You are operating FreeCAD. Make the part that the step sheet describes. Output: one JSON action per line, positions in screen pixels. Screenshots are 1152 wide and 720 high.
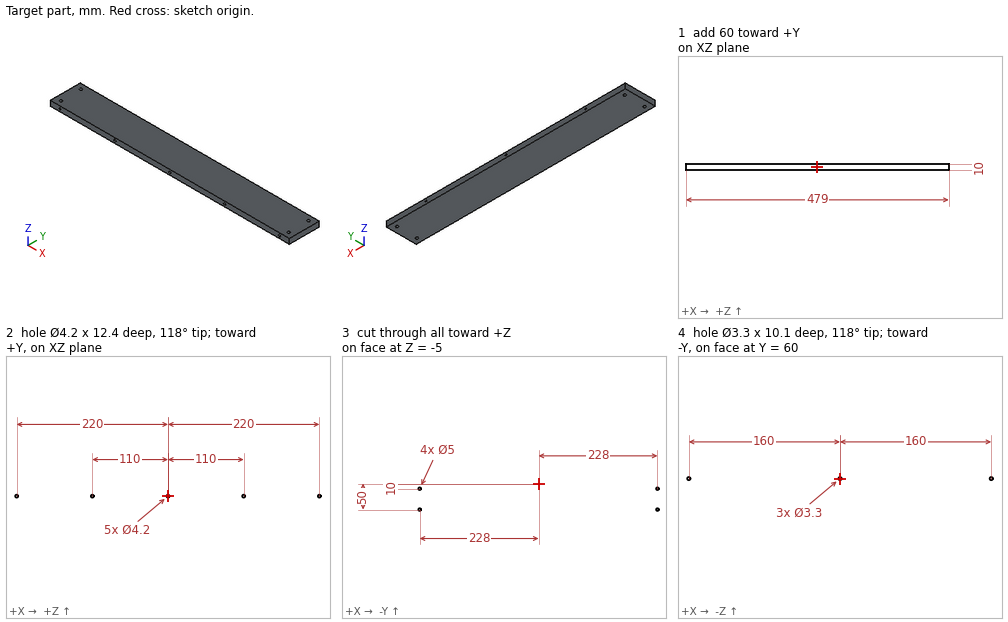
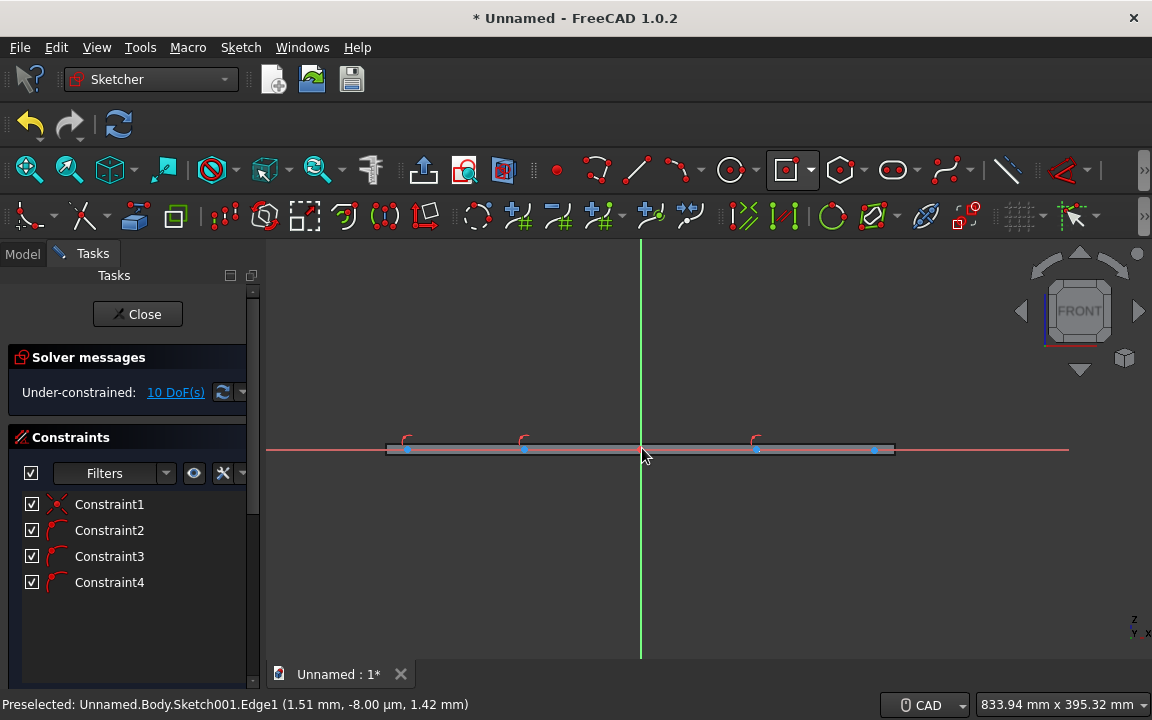
{"action": "scroll", "coordinate": [759, 448], "scroll_direction": "up", "scroll_amount": 11}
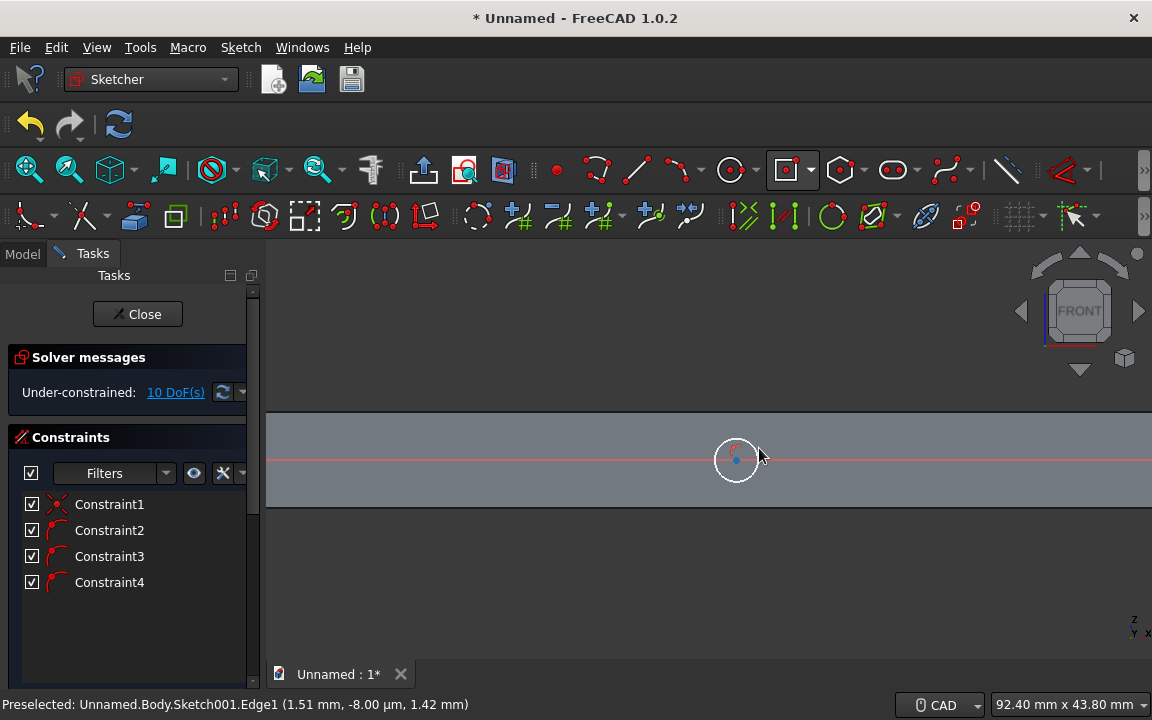
{"action": "left_click", "coordinate": [752, 445]}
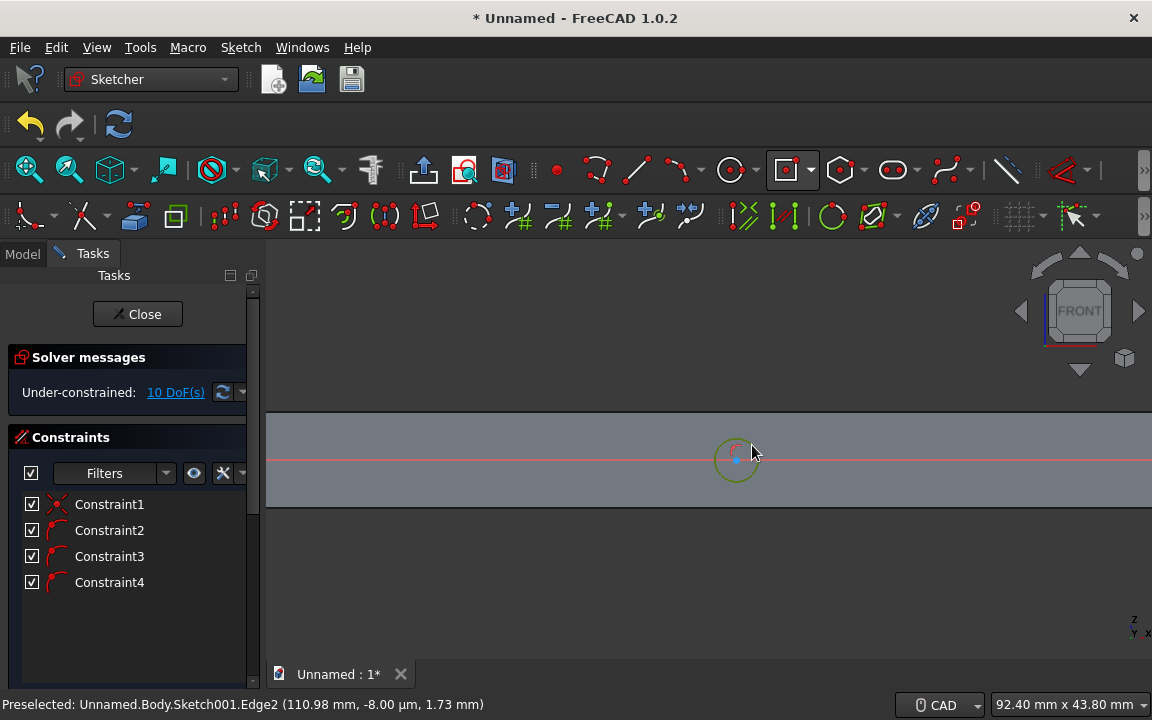
{"action": "scroll", "coordinate": [759, 448], "scroll_direction": "down", "scroll_amount": 11}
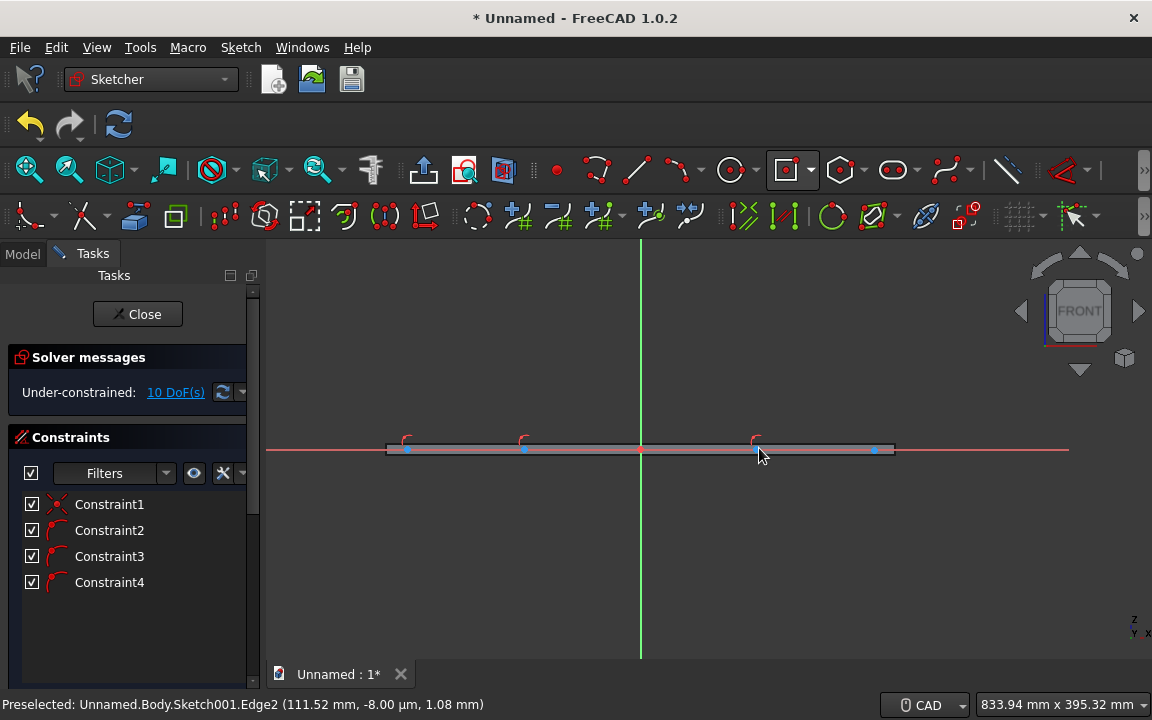
{"action": "scroll", "coordinate": [875, 450], "scroll_direction": "up", "scroll_amount": 13}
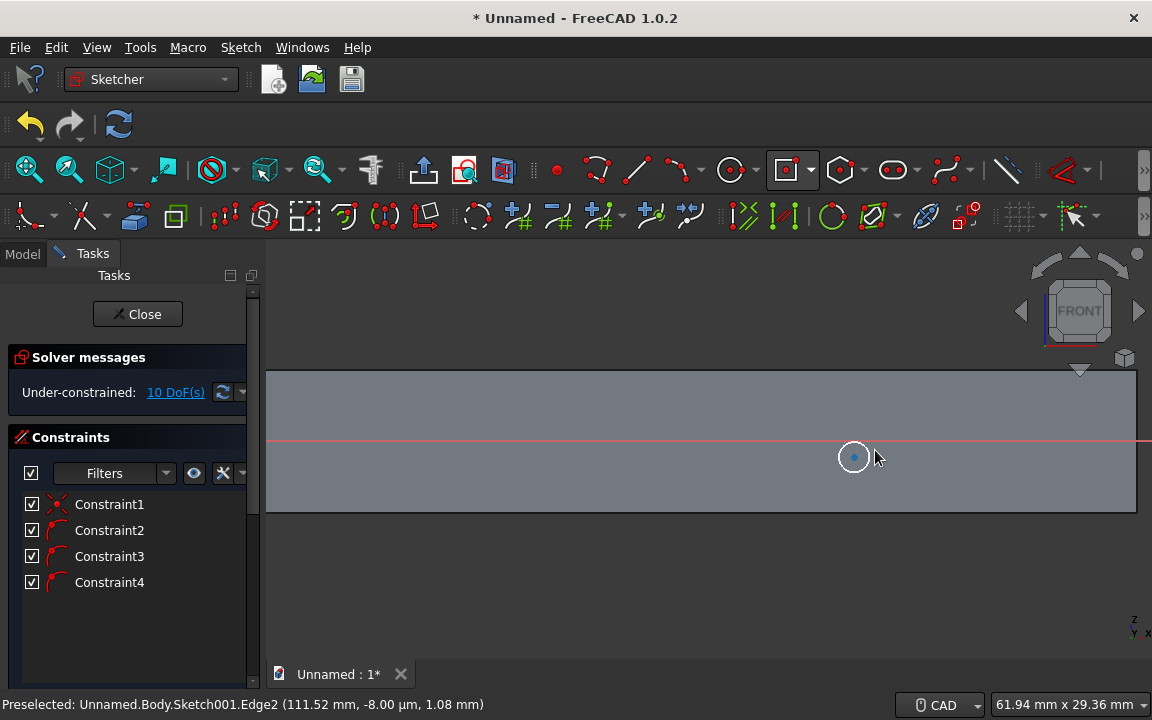
{"action": "left_click", "coordinate": [865, 446]}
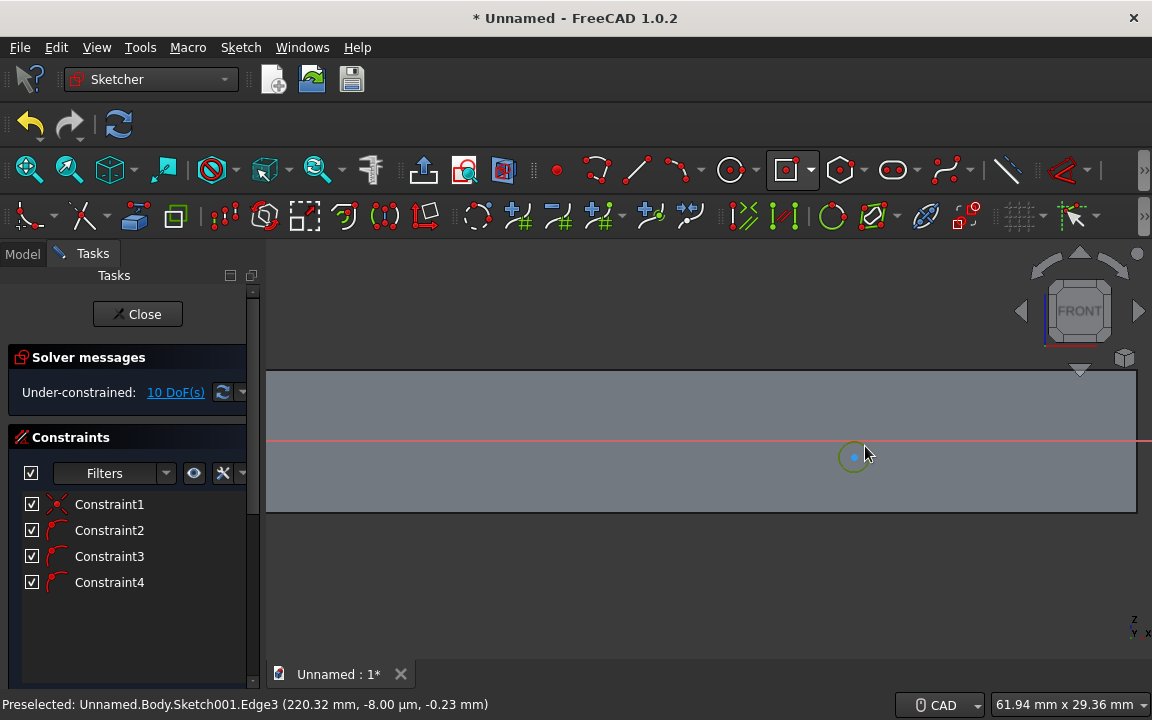
{"action": "scroll", "coordinate": [876, 450], "scroll_direction": "down", "scroll_amount": 13}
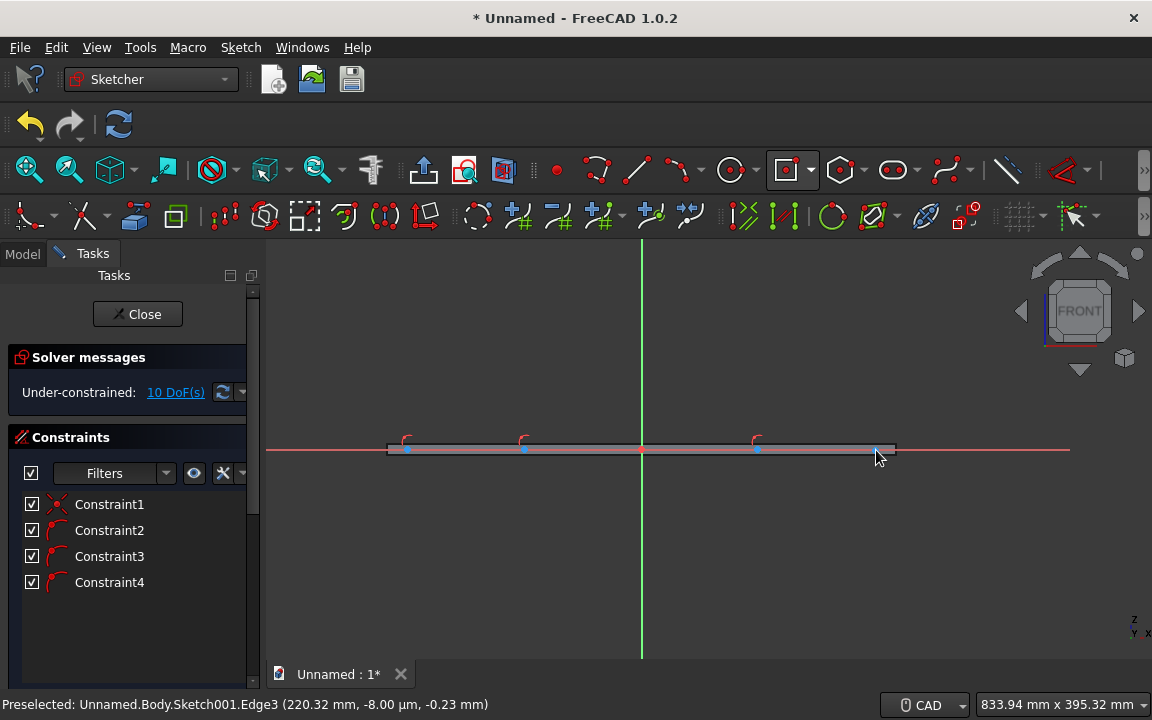
{"action": "scroll", "coordinate": [409, 448], "scroll_direction": "up", "scroll_amount": 12}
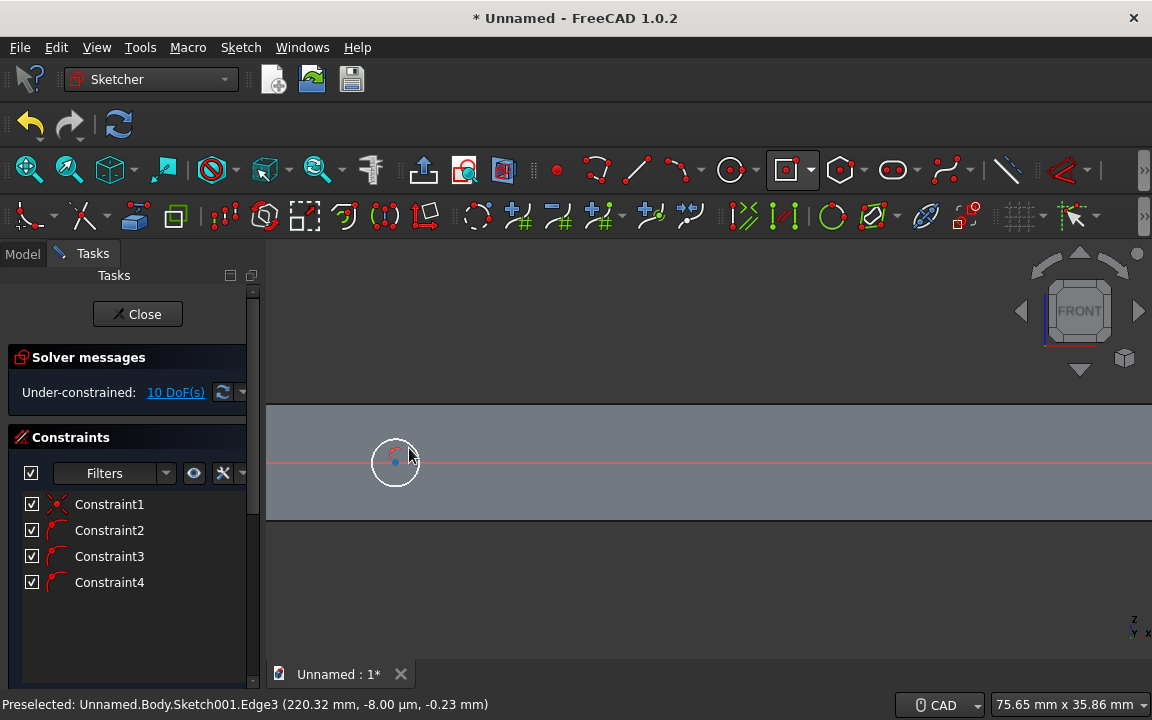
{"action": "left_click", "coordinate": [412, 446]}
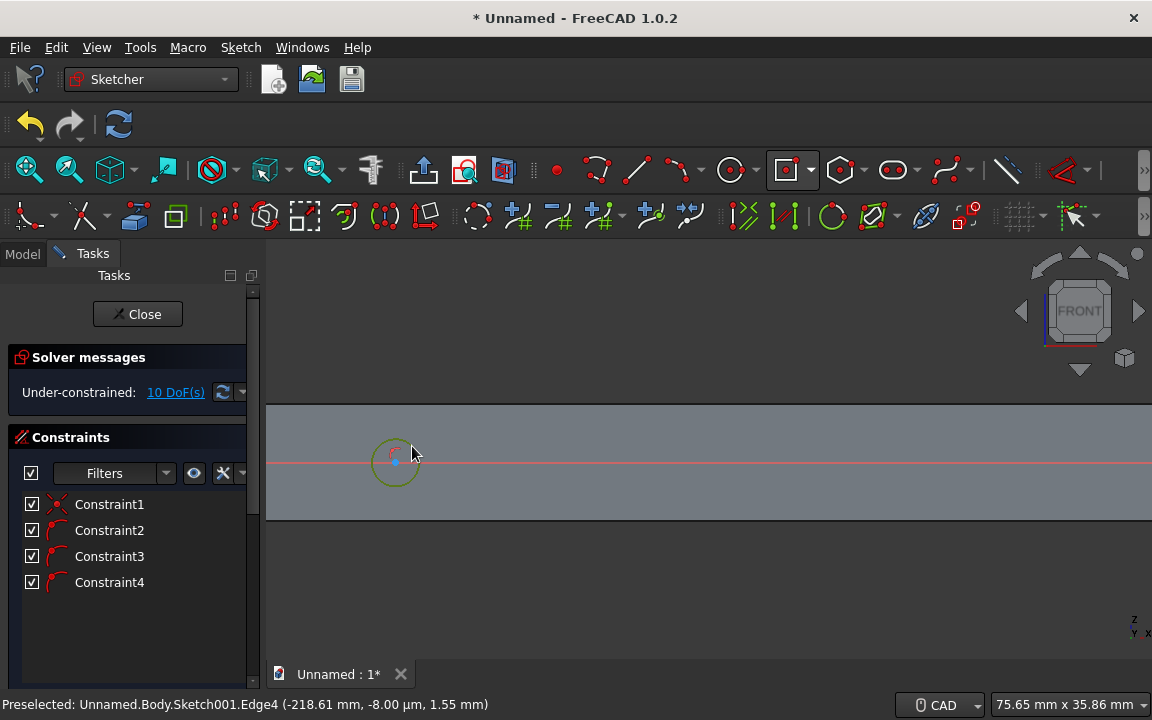
{"action": "scroll", "coordinate": [408, 448], "scroll_direction": "down", "scroll_amount": 12}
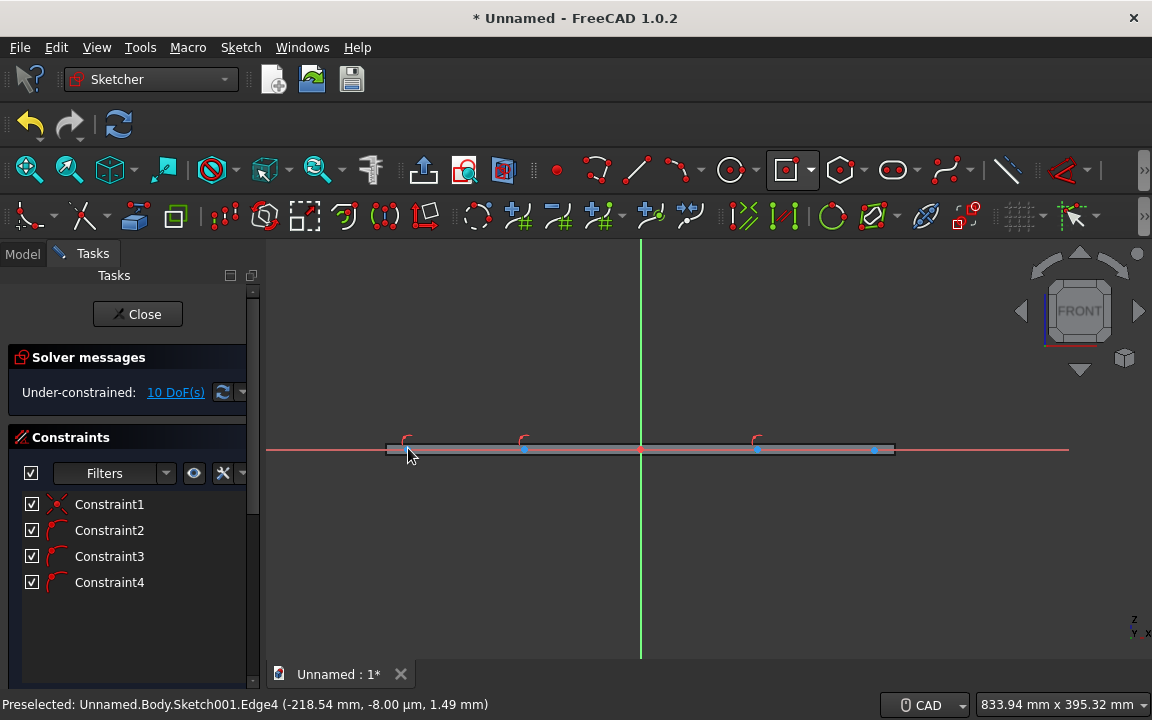
{"action": "scroll", "coordinate": [525, 448], "scroll_direction": "up", "scroll_amount": 12}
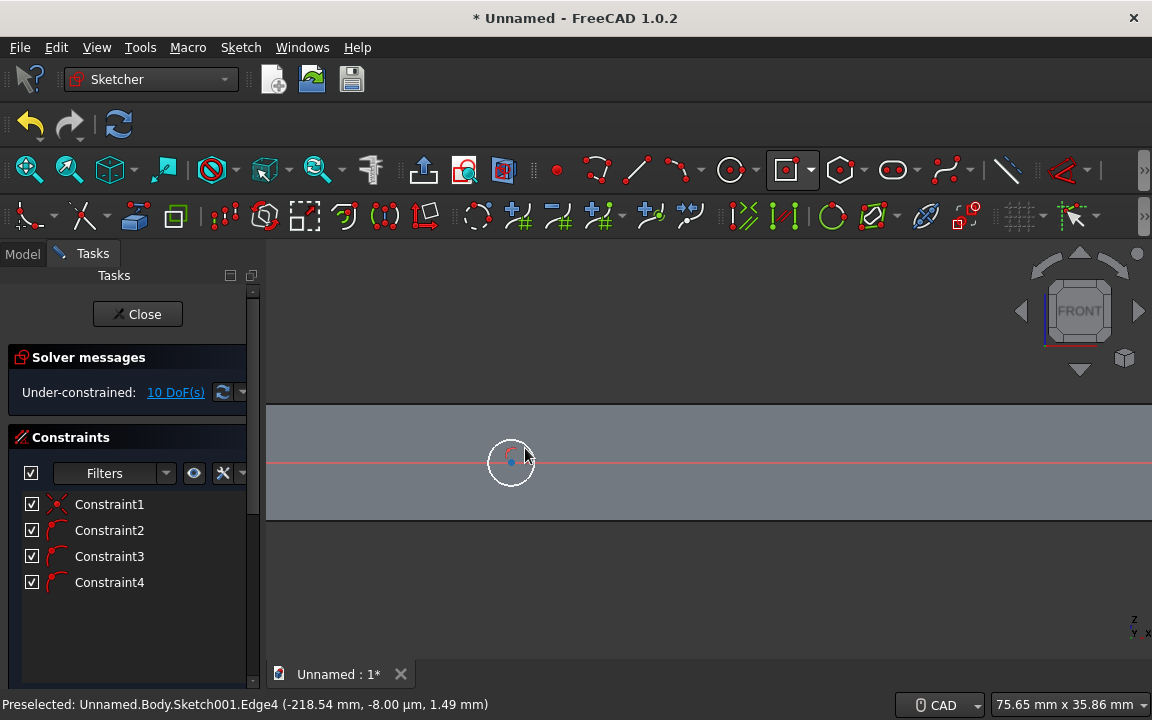
{"action": "left_click", "coordinate": [527, 447]}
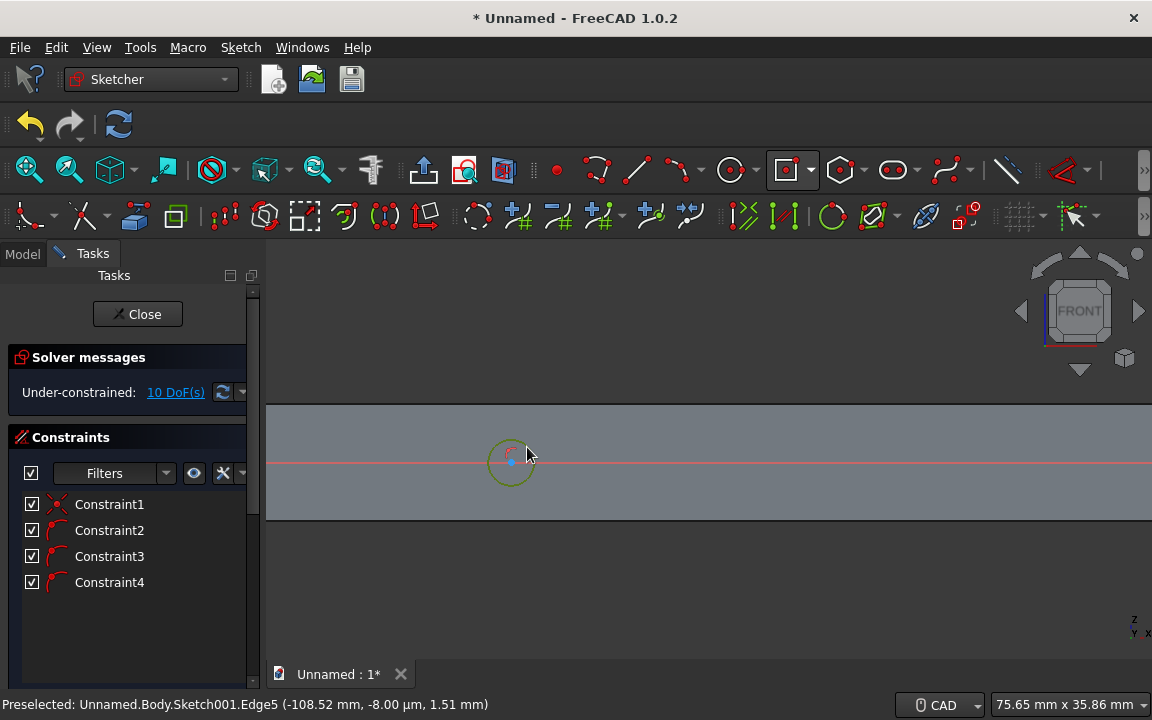
{"action": "key", "text": "e"}